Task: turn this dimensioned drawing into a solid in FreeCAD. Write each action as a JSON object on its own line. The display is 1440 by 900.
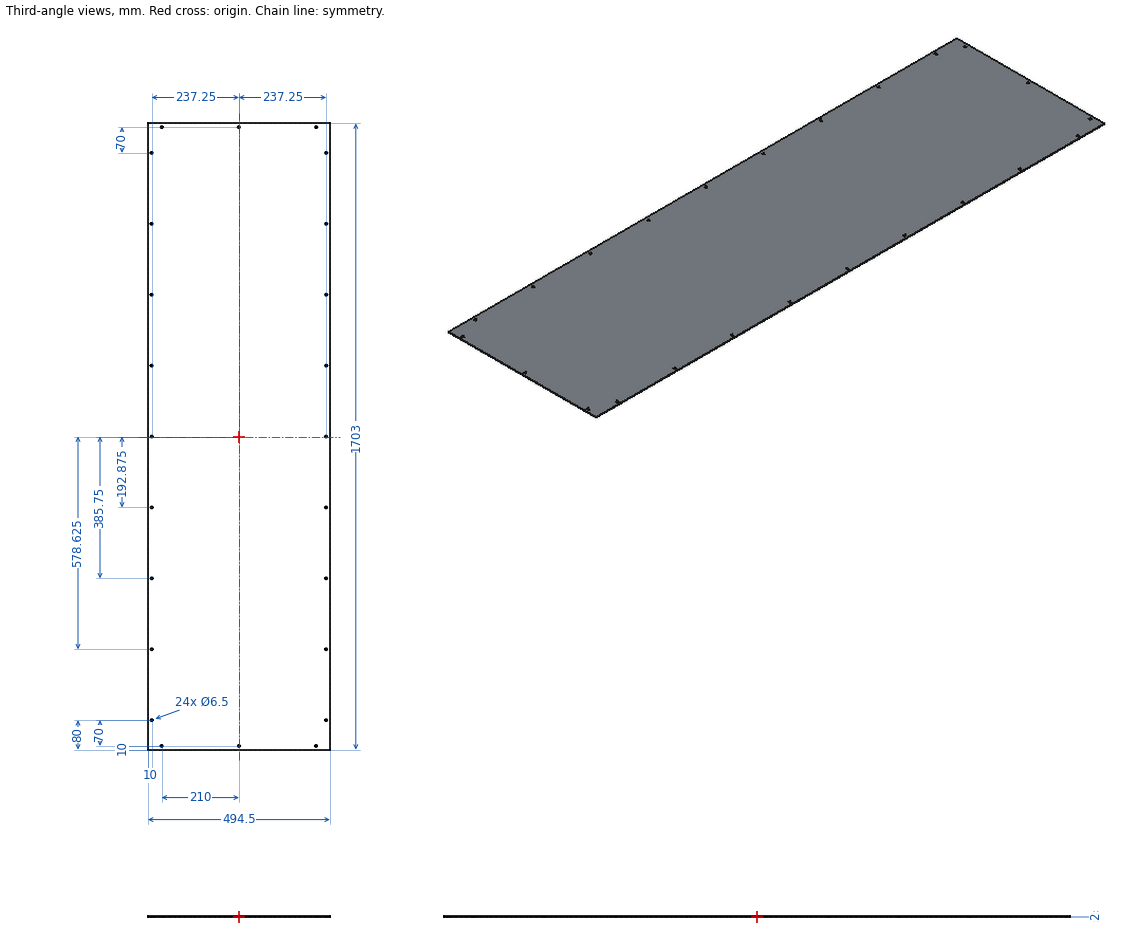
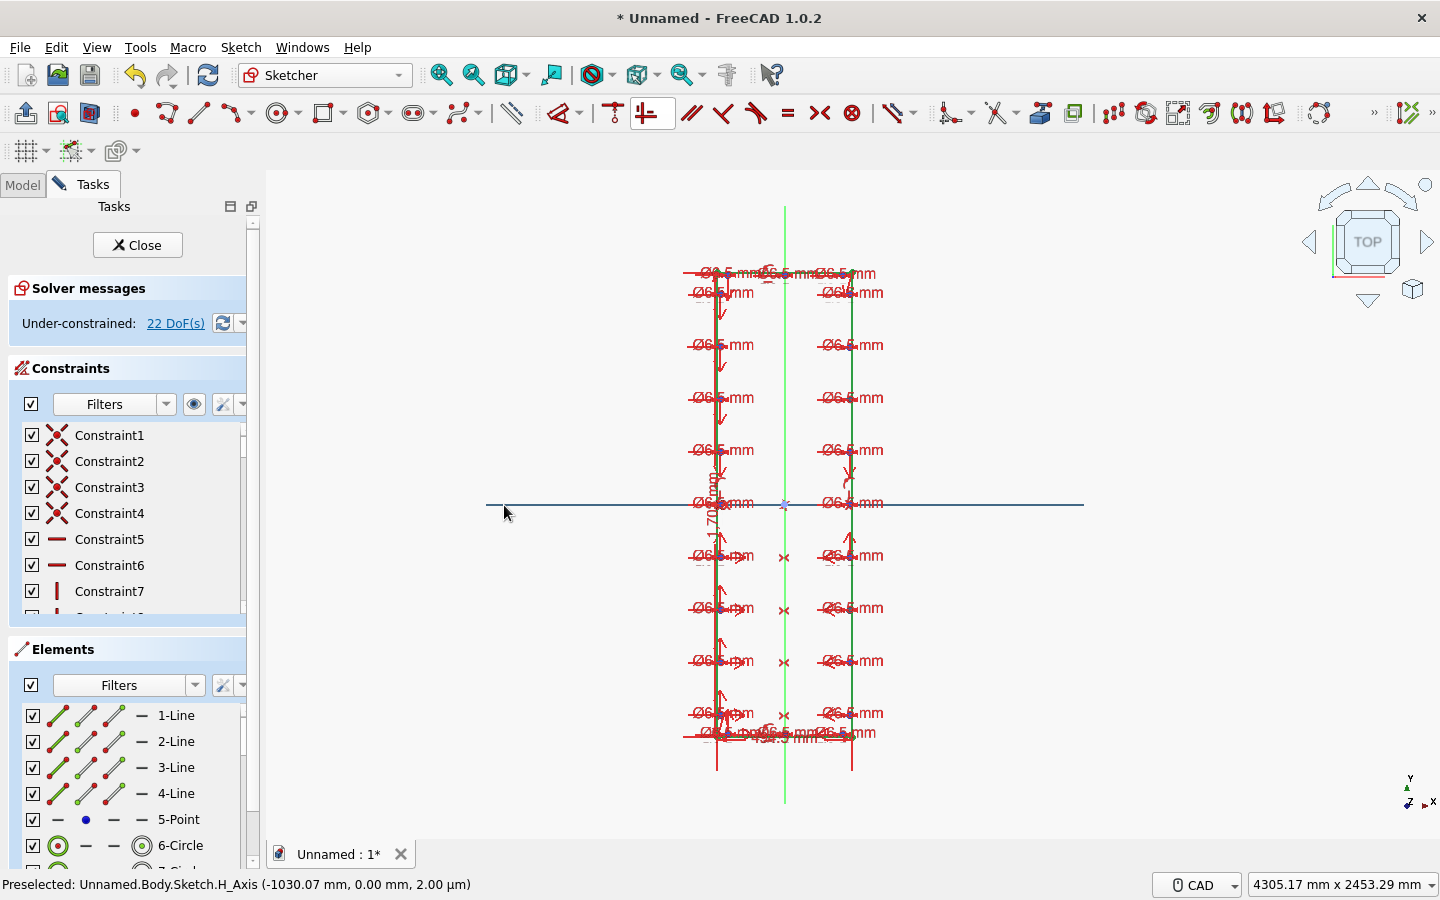
{"action": "left_click", "coordinate": [820, 114]}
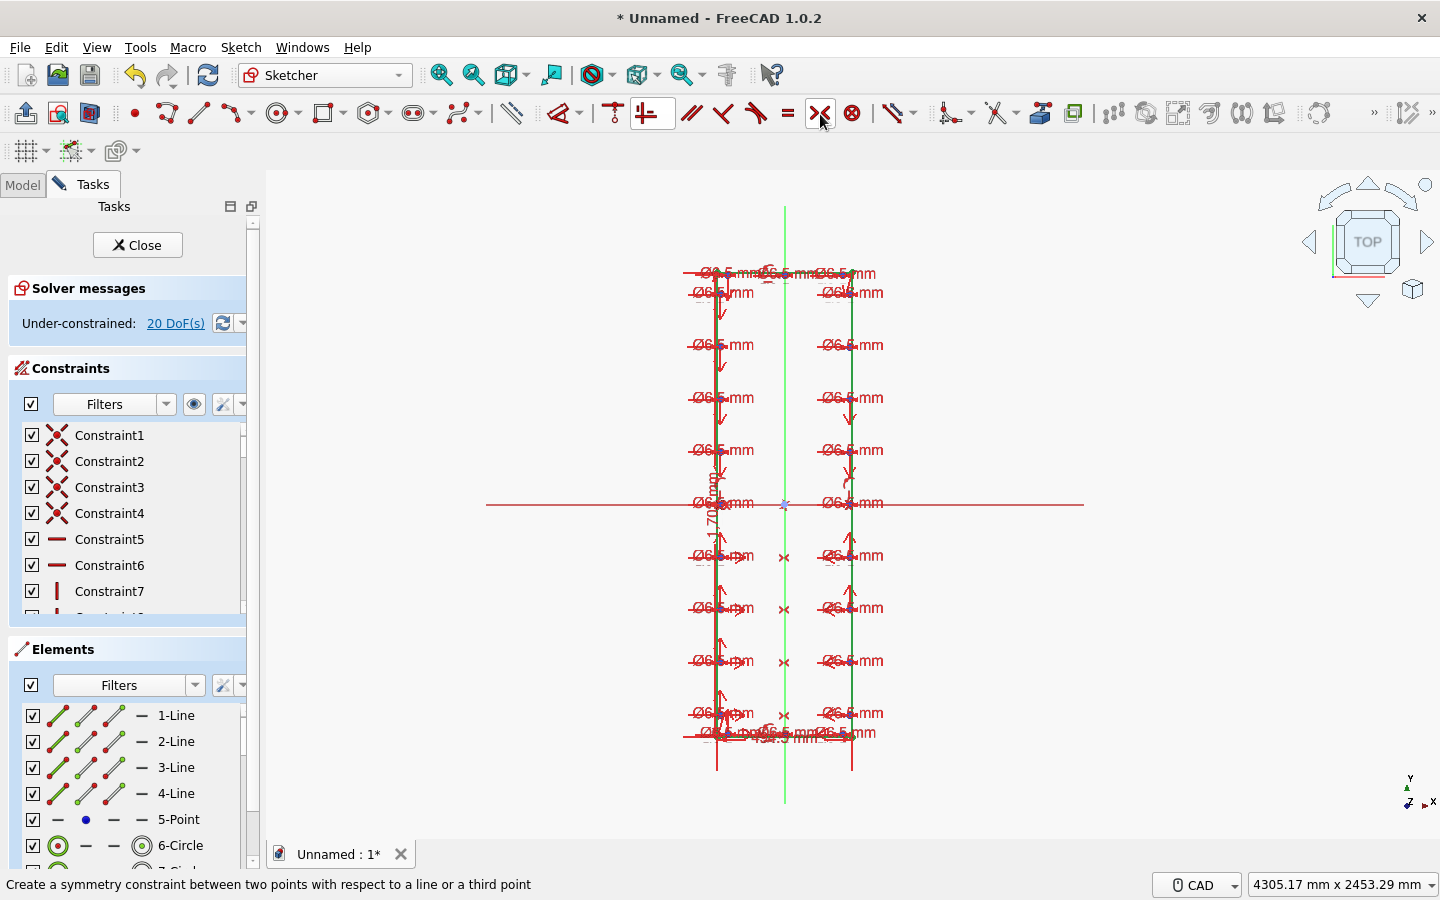
{"action": "left_click", "coordinate": [850, 663]}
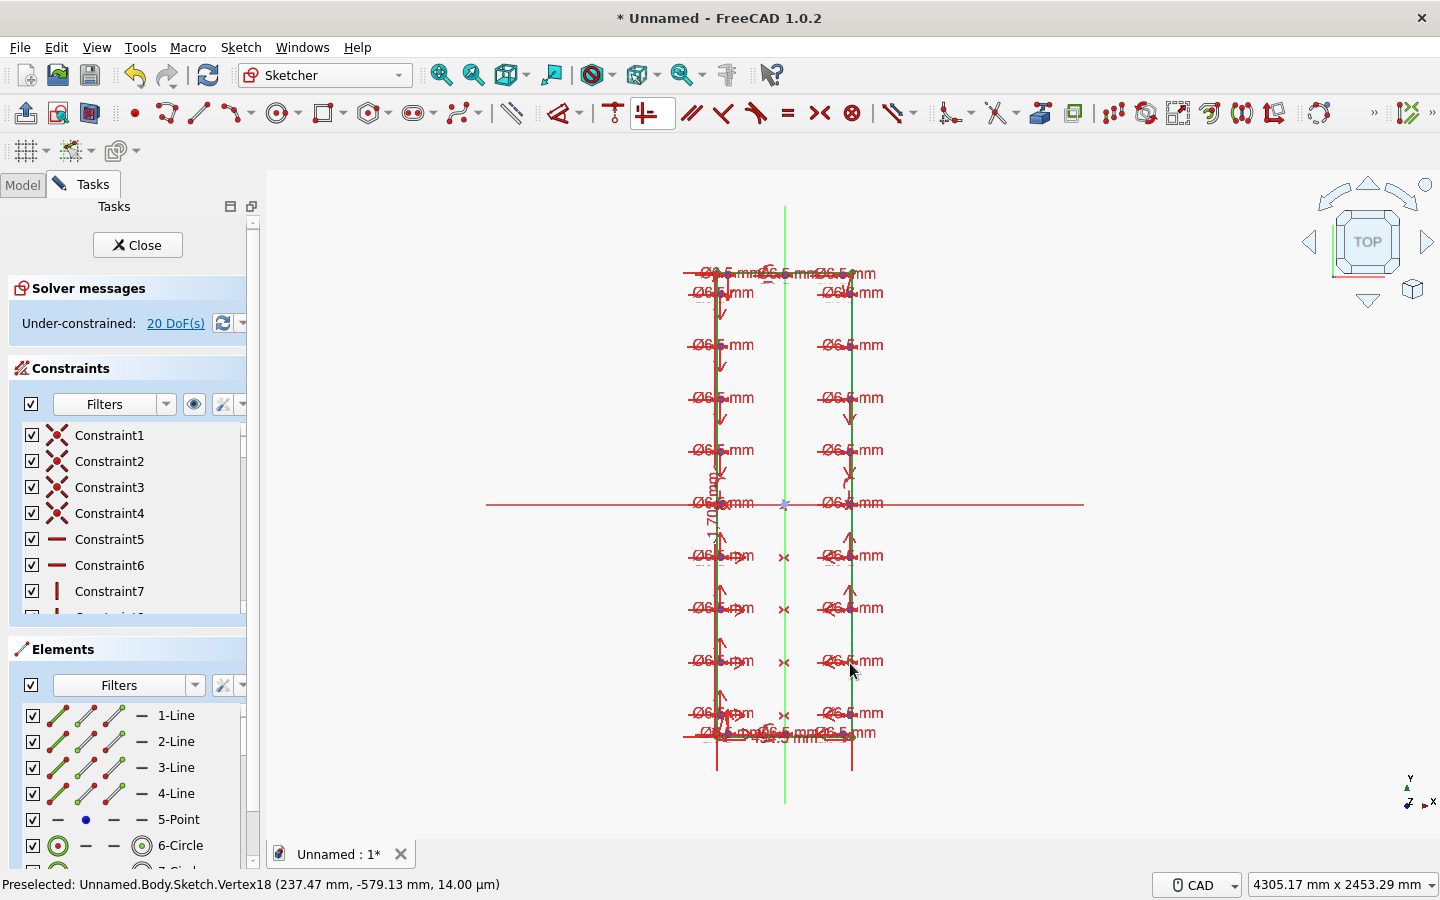
{"action": "left_click", "coordinate": [850, 347]}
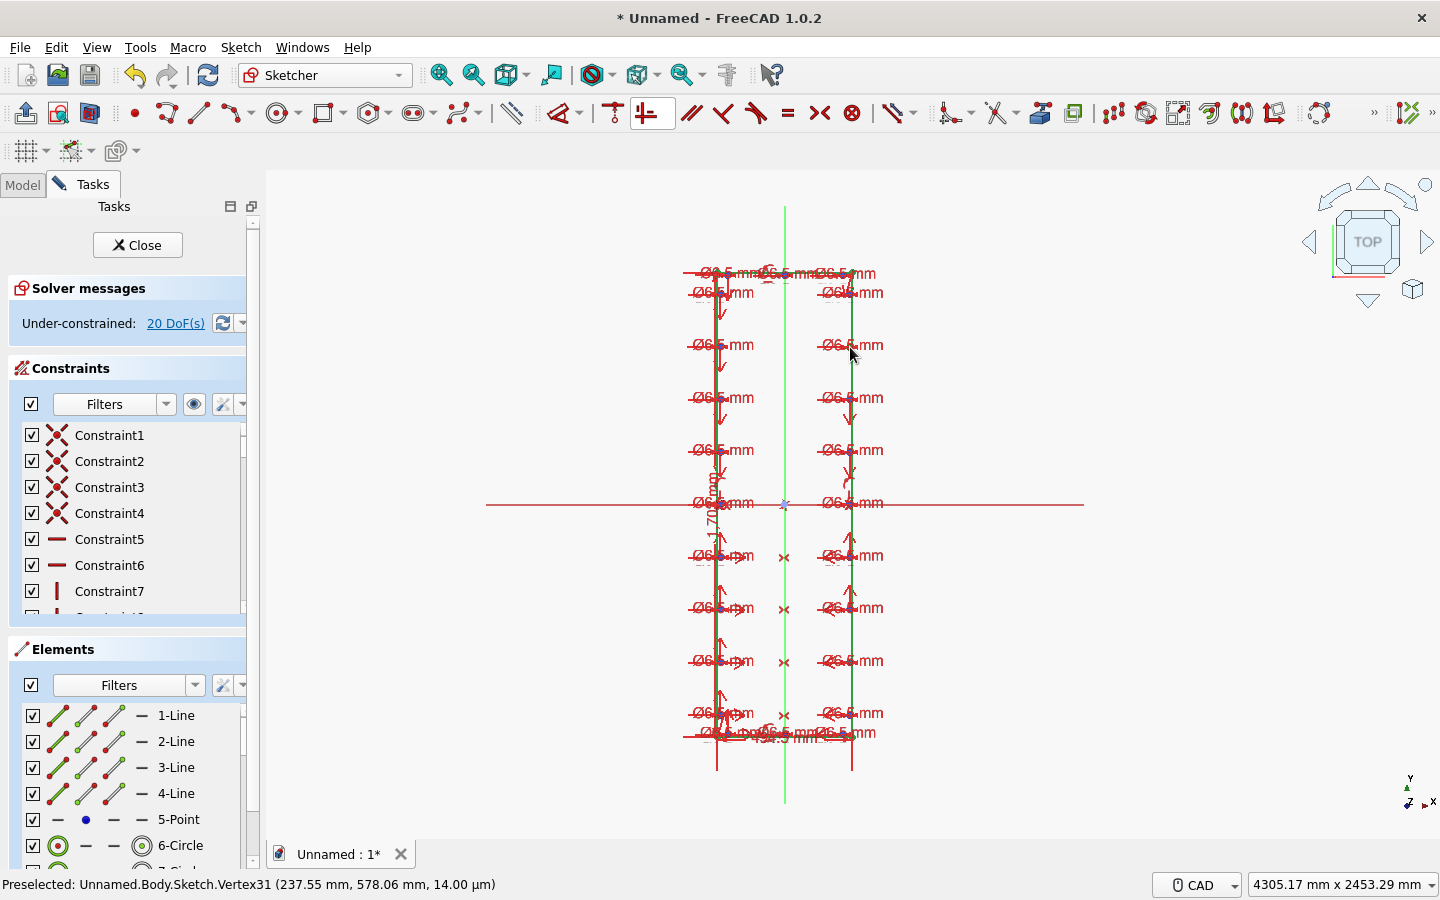
{"action": "left_click", "coordinate": [504, 505]}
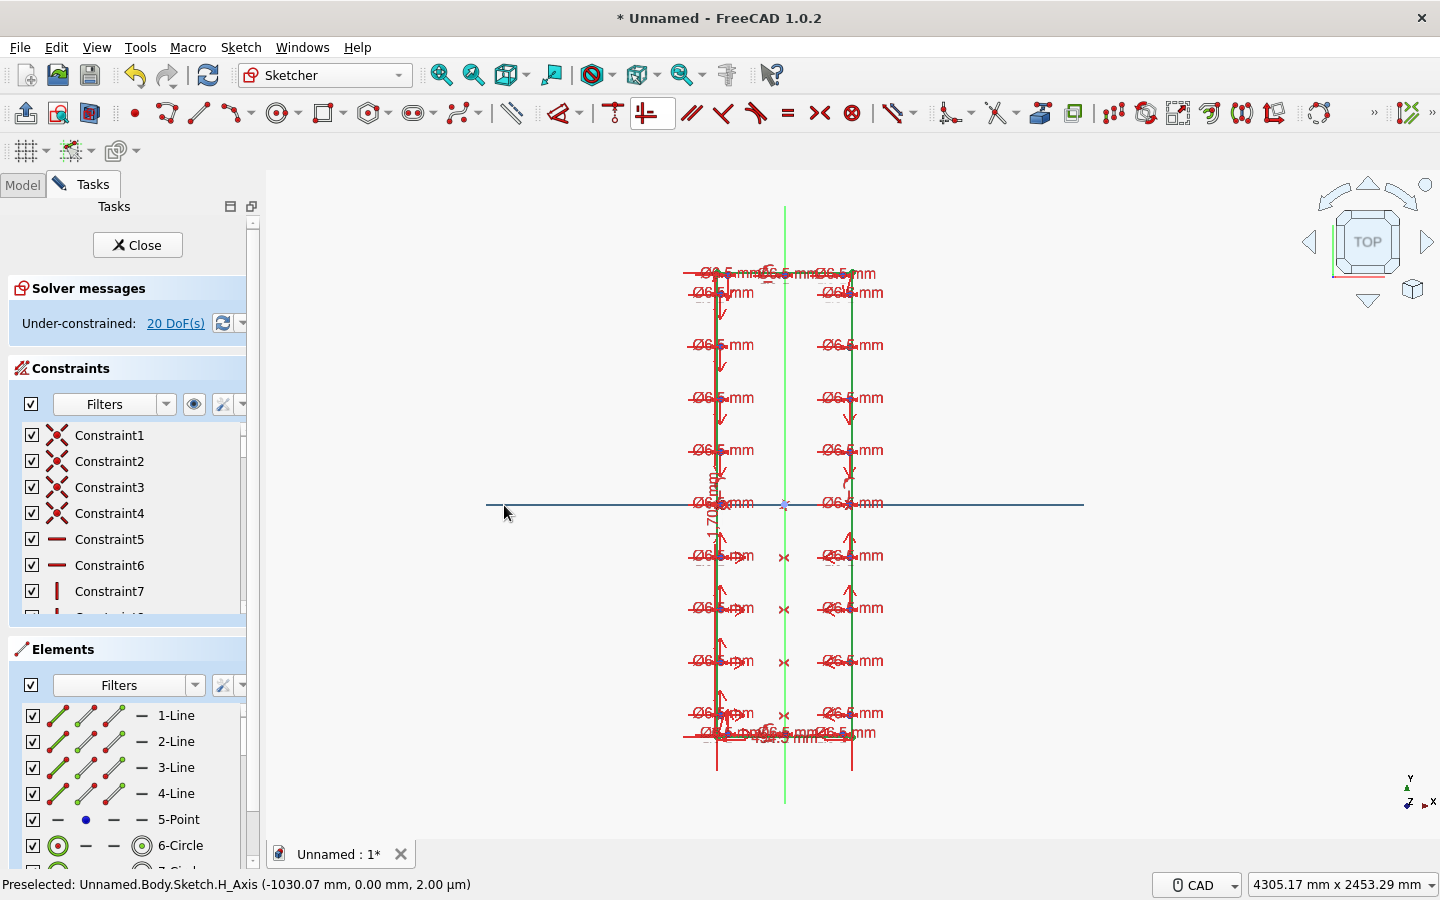
{"action": "left_click", "coordinate": [820, 114]}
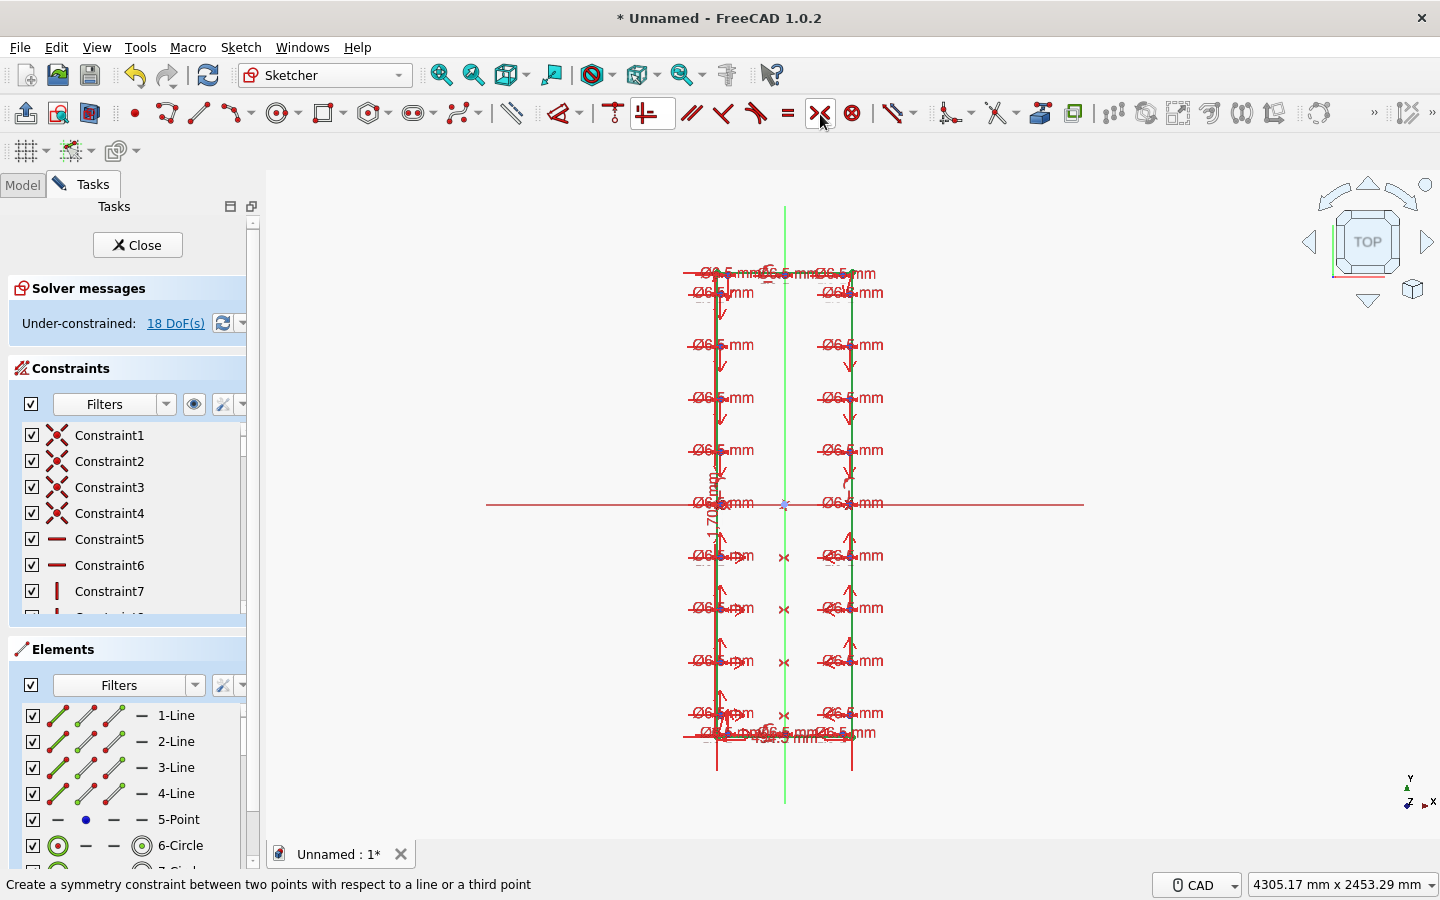
{"action": "left_click", "coordinate": [842, 735]}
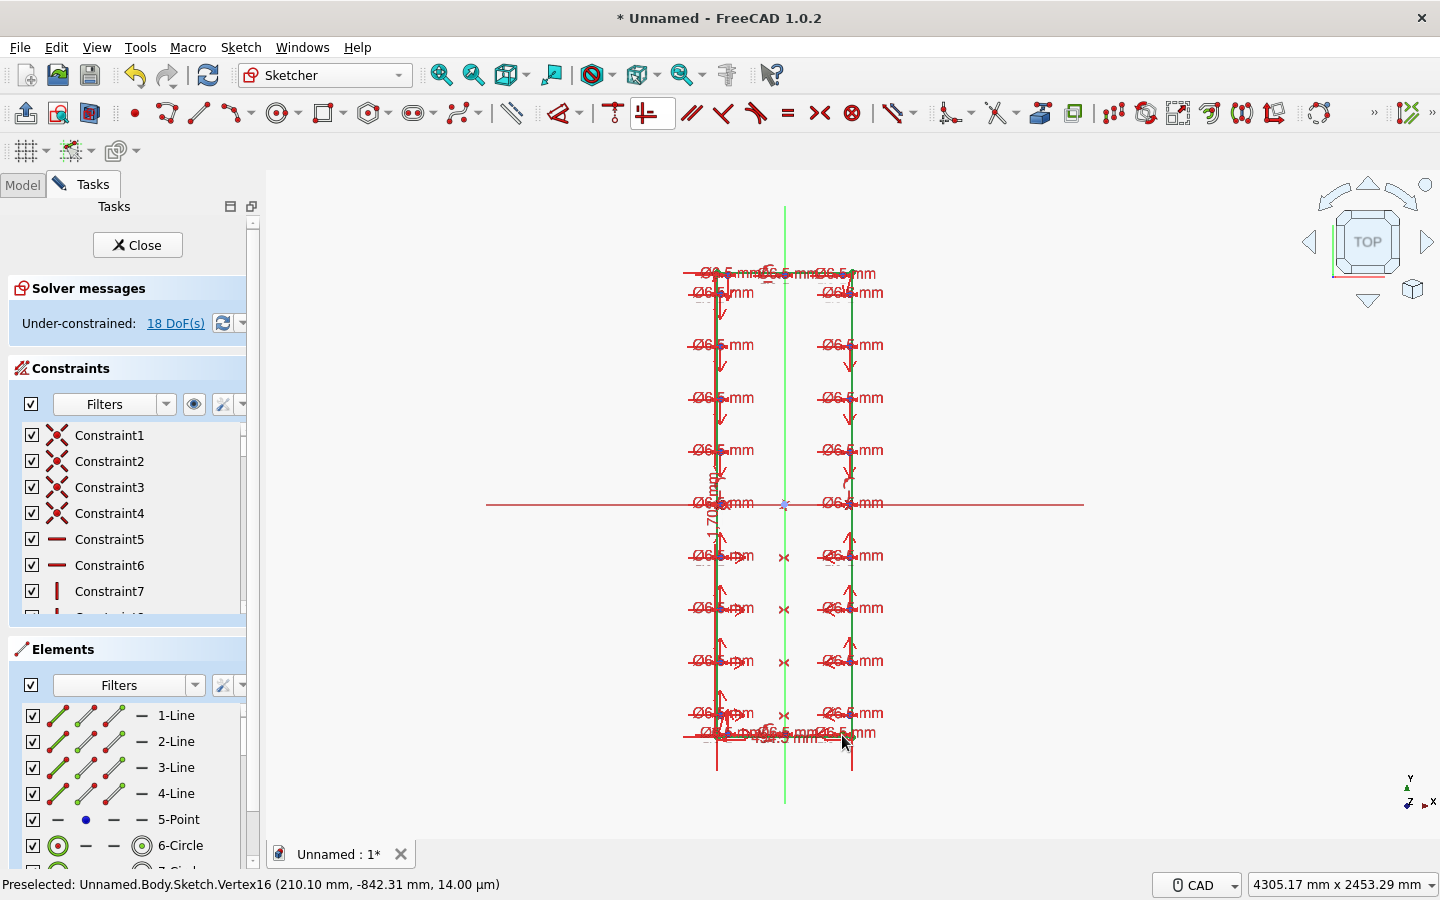
{"action": "left_click", "coordinate": [842, 276]}